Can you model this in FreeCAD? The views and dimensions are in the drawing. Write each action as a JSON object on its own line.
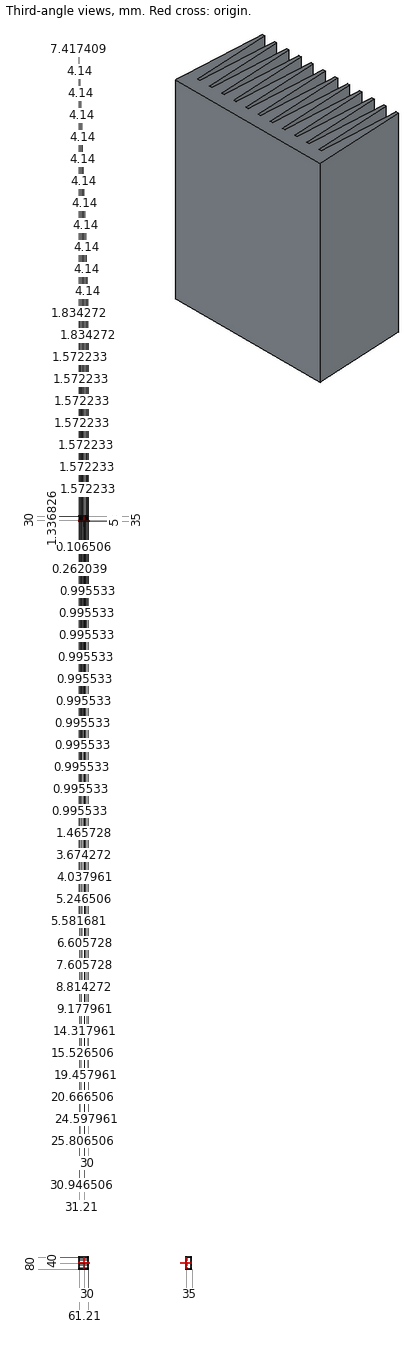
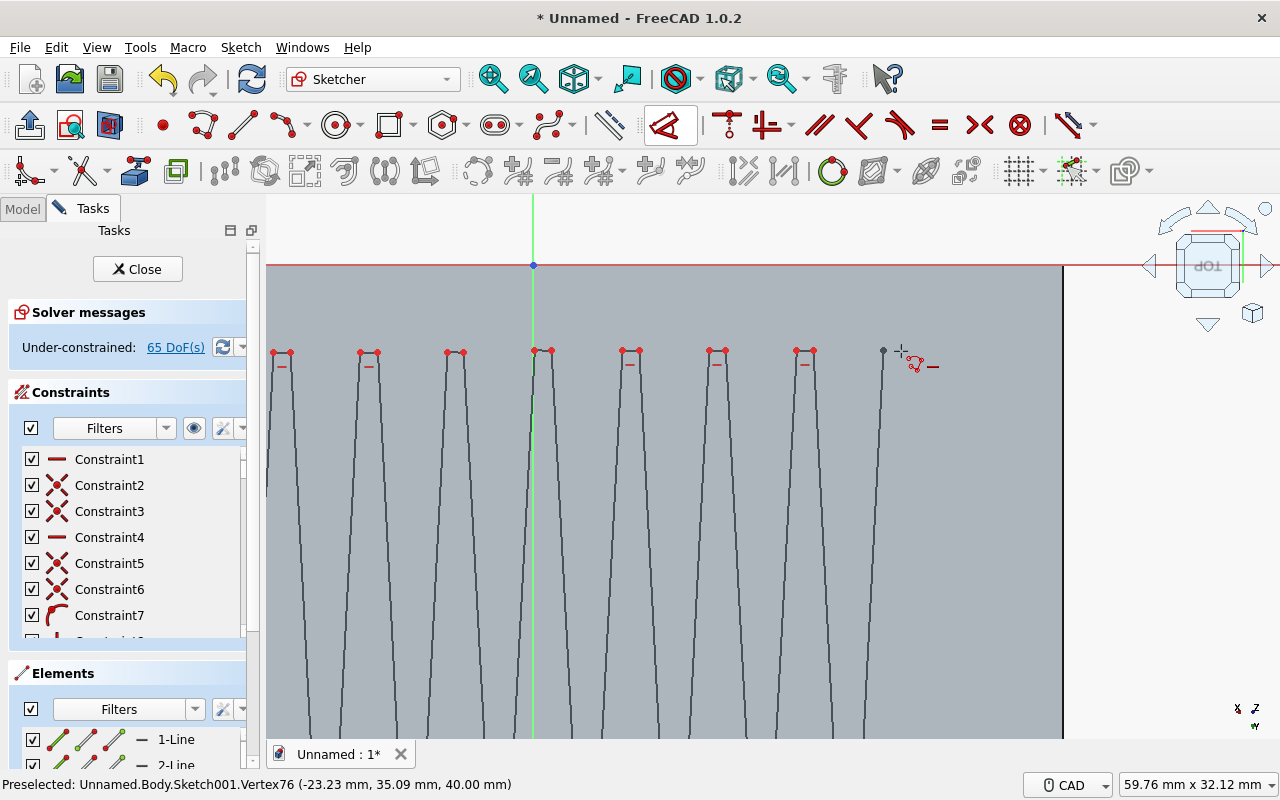
{"action": "left_click", "coordinate": [901, 350]}
{"action": "left_click", "coordinate": [883, 351]}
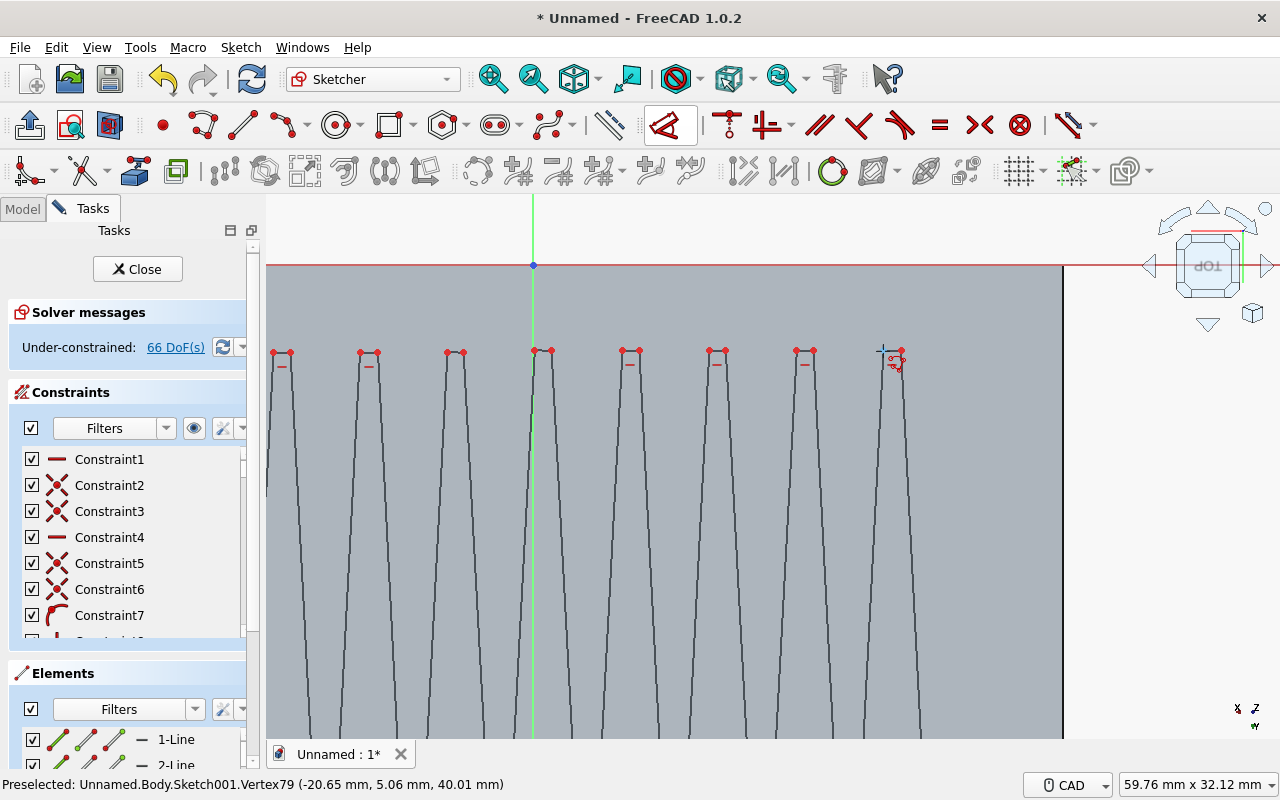
{"action": "left_click", "coordinate": [971, 350]}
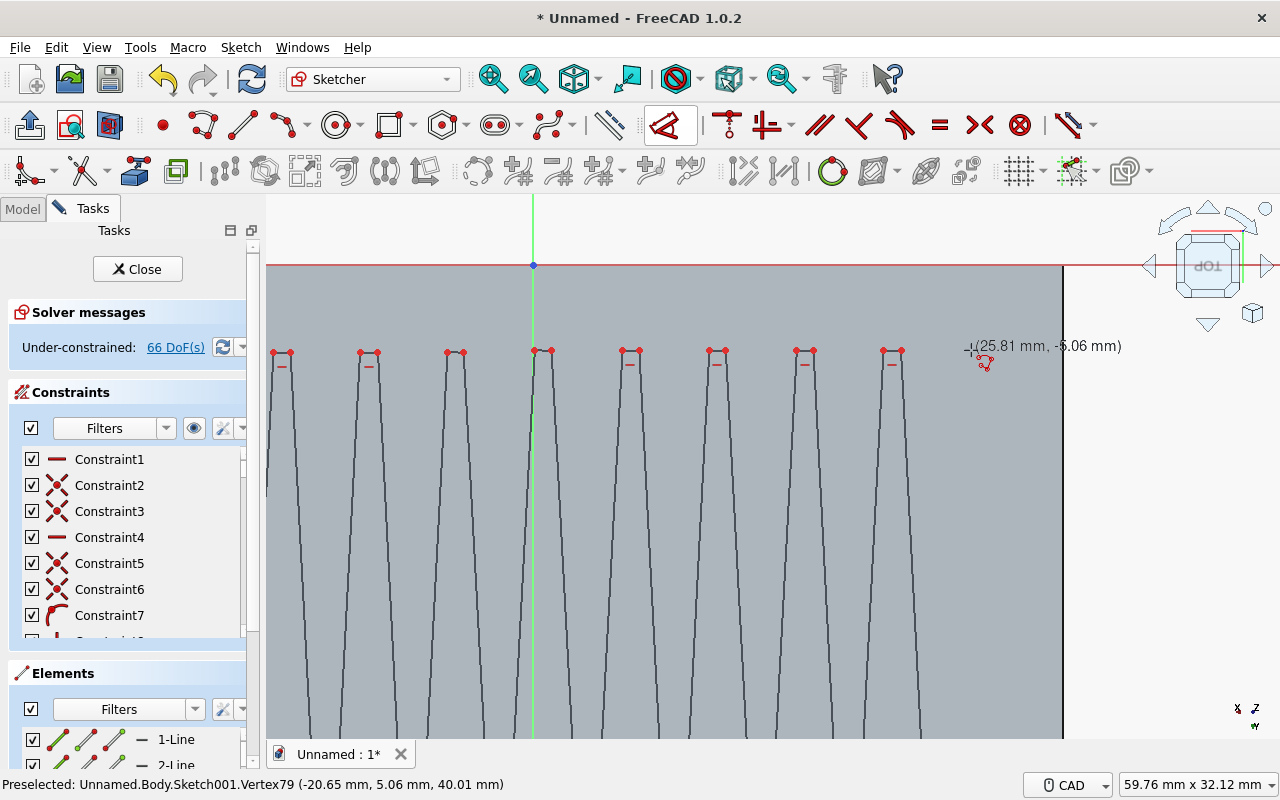
{"action": "scroll", "coordinate": [901, 350], "scroll_direction": "down", "scroll_amount": 3}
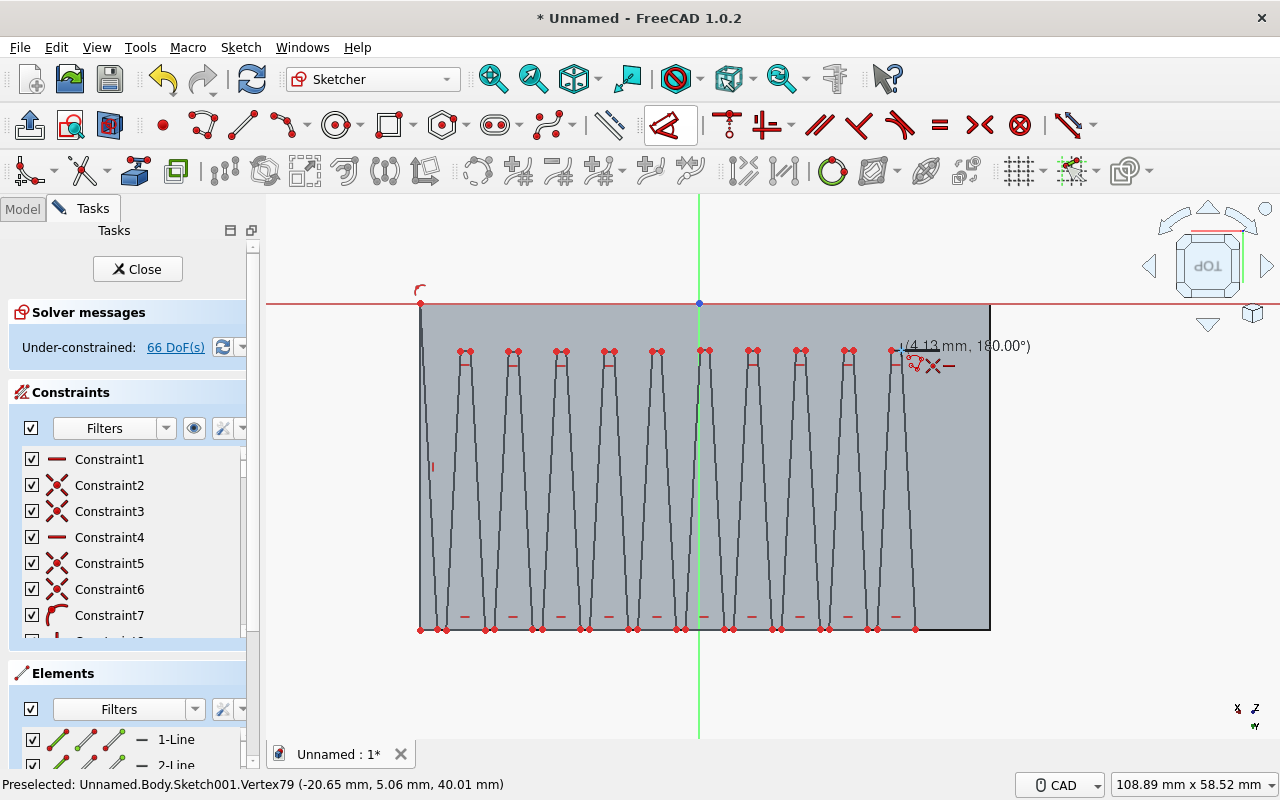
{"action": "scroll", "coordinate": [925, 630], "scroll_direction": "up", "scroll_amount": 3}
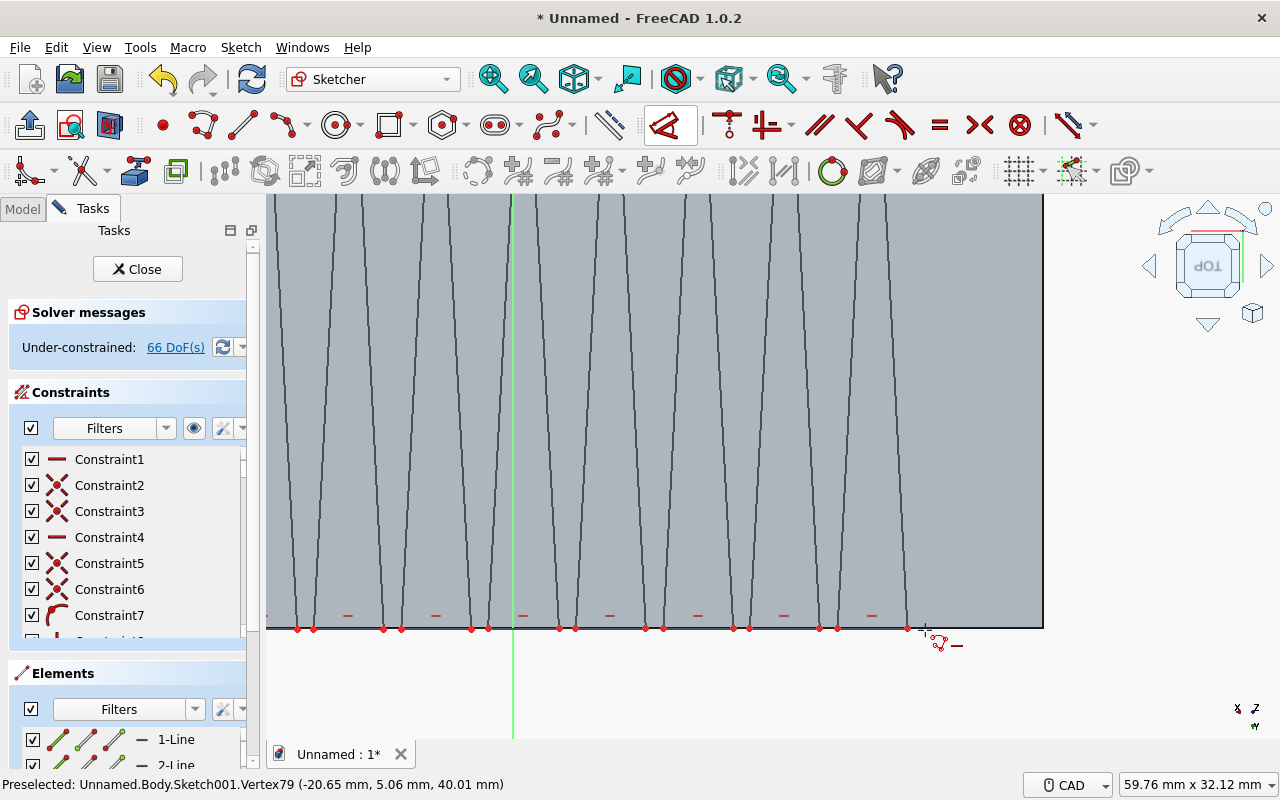
{"action": "left_click", "coordinate": [925, 628]}
{"action": "left_click", "coordinate": [995, 628]}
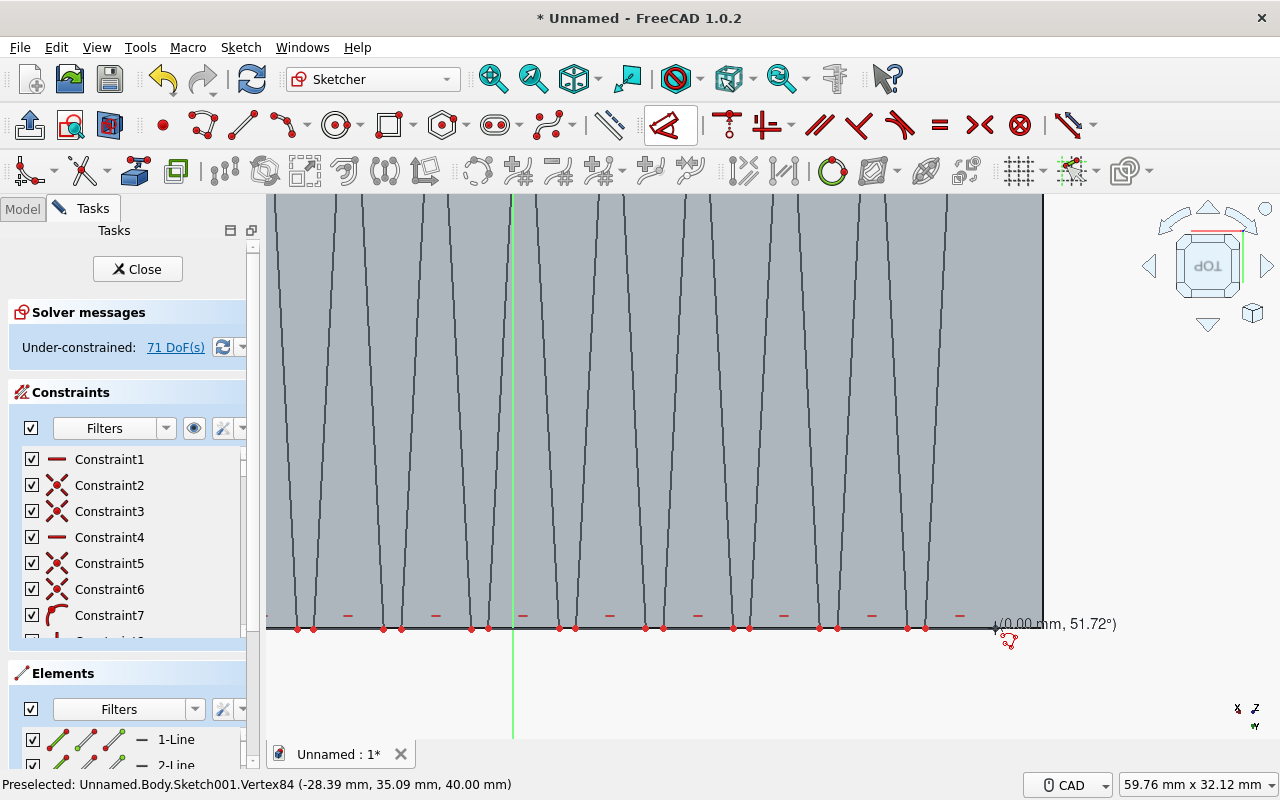
{"action": "scroll", "coordinate": [925, 631], "scroll_direction": "down", "scroll_amount": 3}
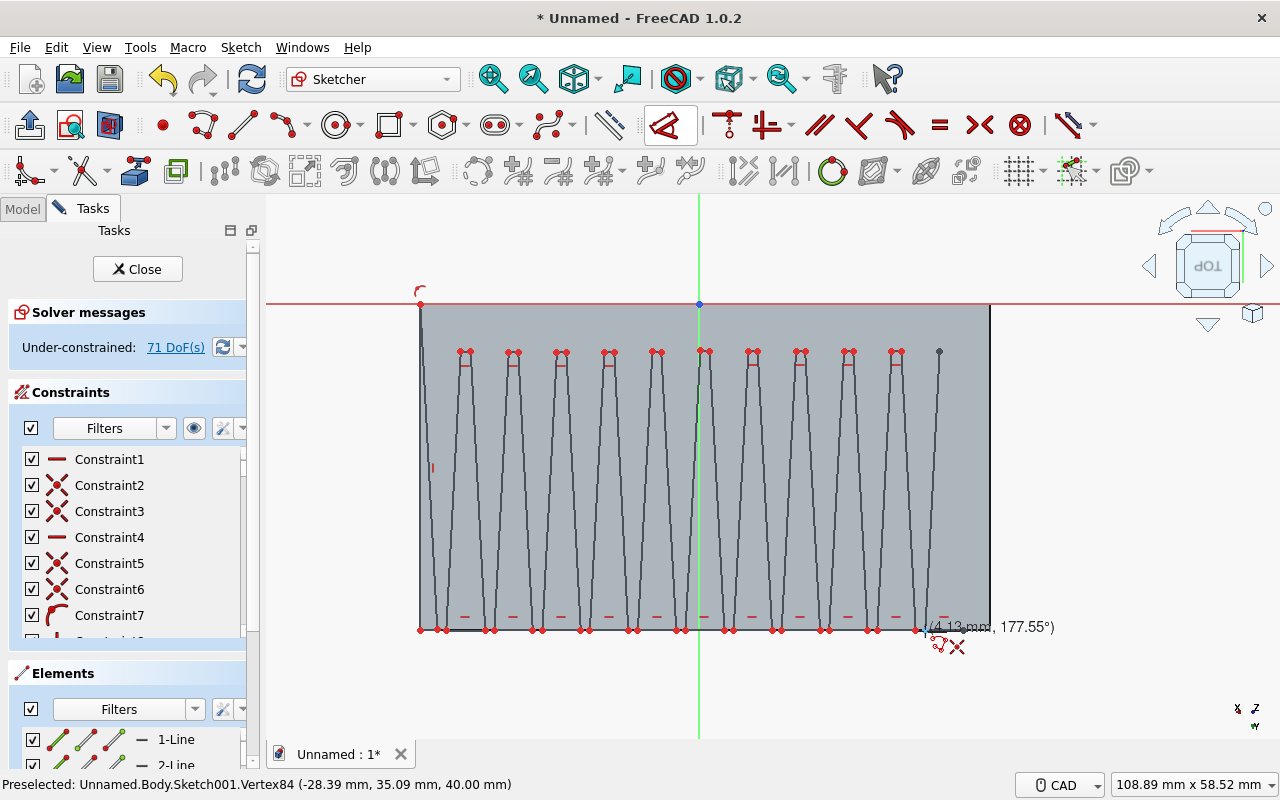
{"action": "scroll", "coordinate": [949, 351], "scroll_direction": "up", "scroll_amount": 3}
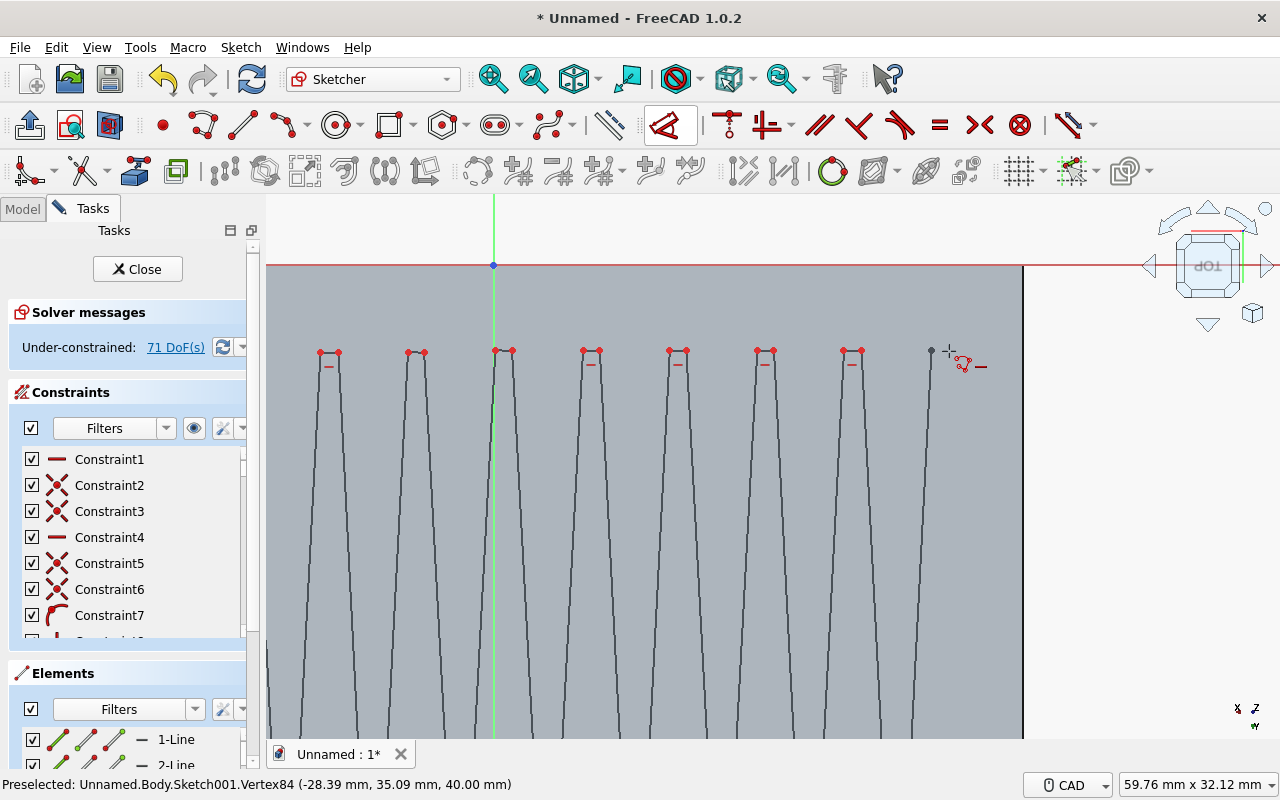
{"action": "left_click", "coordinate": [948, 350]}
{"action": "left_click", "coordinate": [931, 351]}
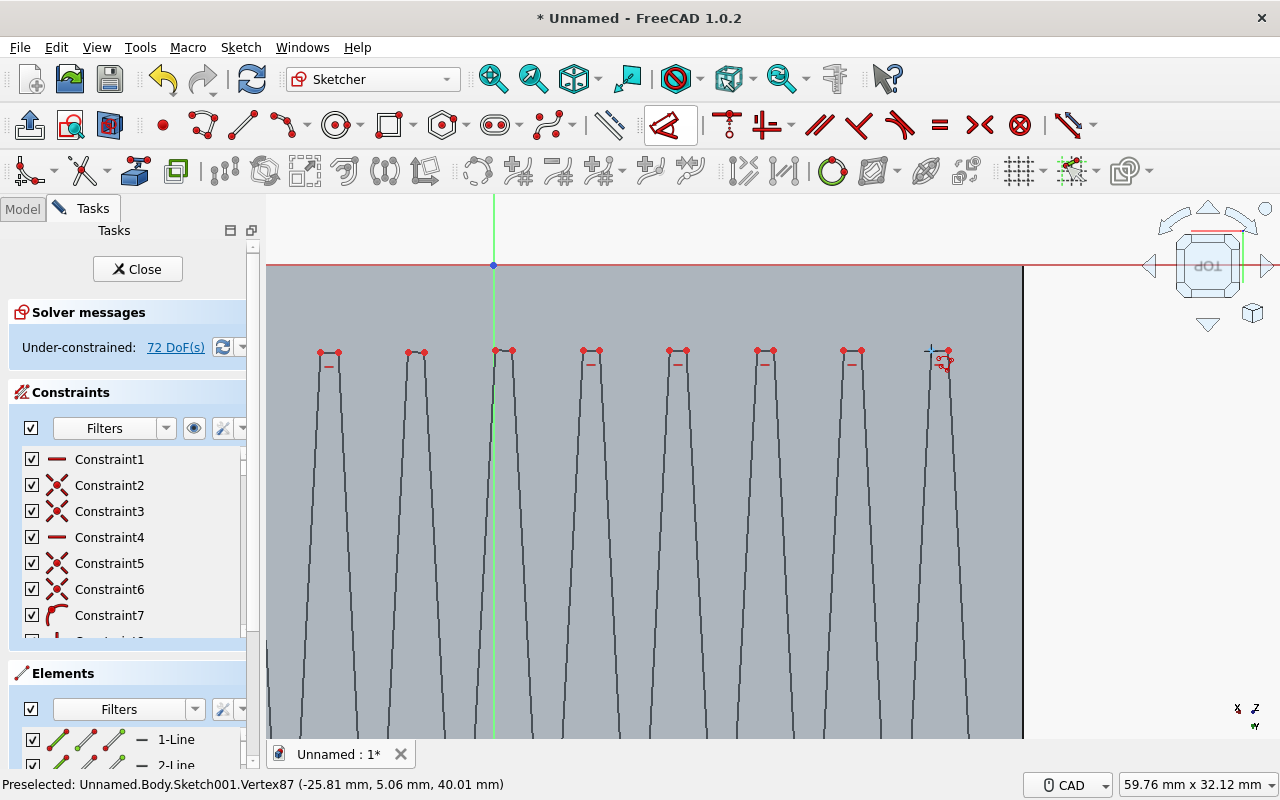
{"action": "left_click", "coordinate": [1019, 350]}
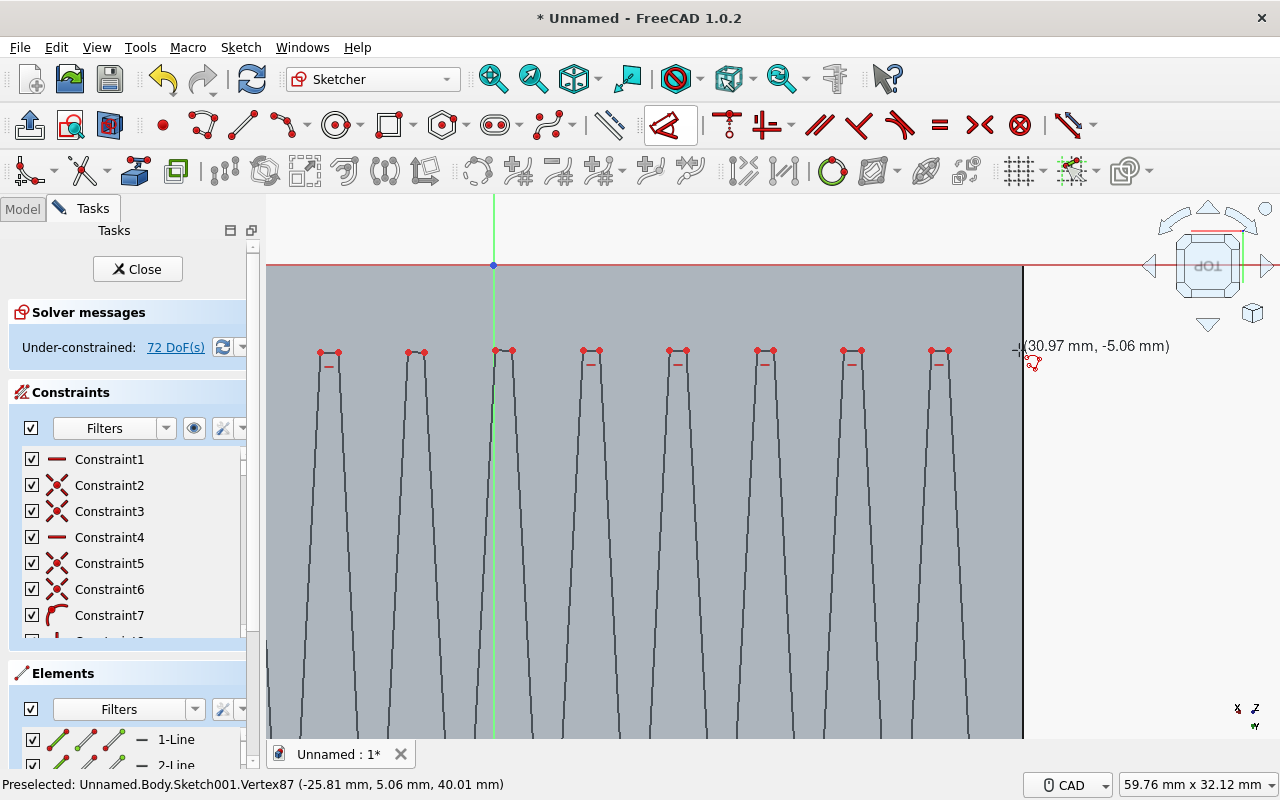
{"action": "scroll", "coordinate": [949, 350], "scroll_direction": "down", "scroll_amount": 3}